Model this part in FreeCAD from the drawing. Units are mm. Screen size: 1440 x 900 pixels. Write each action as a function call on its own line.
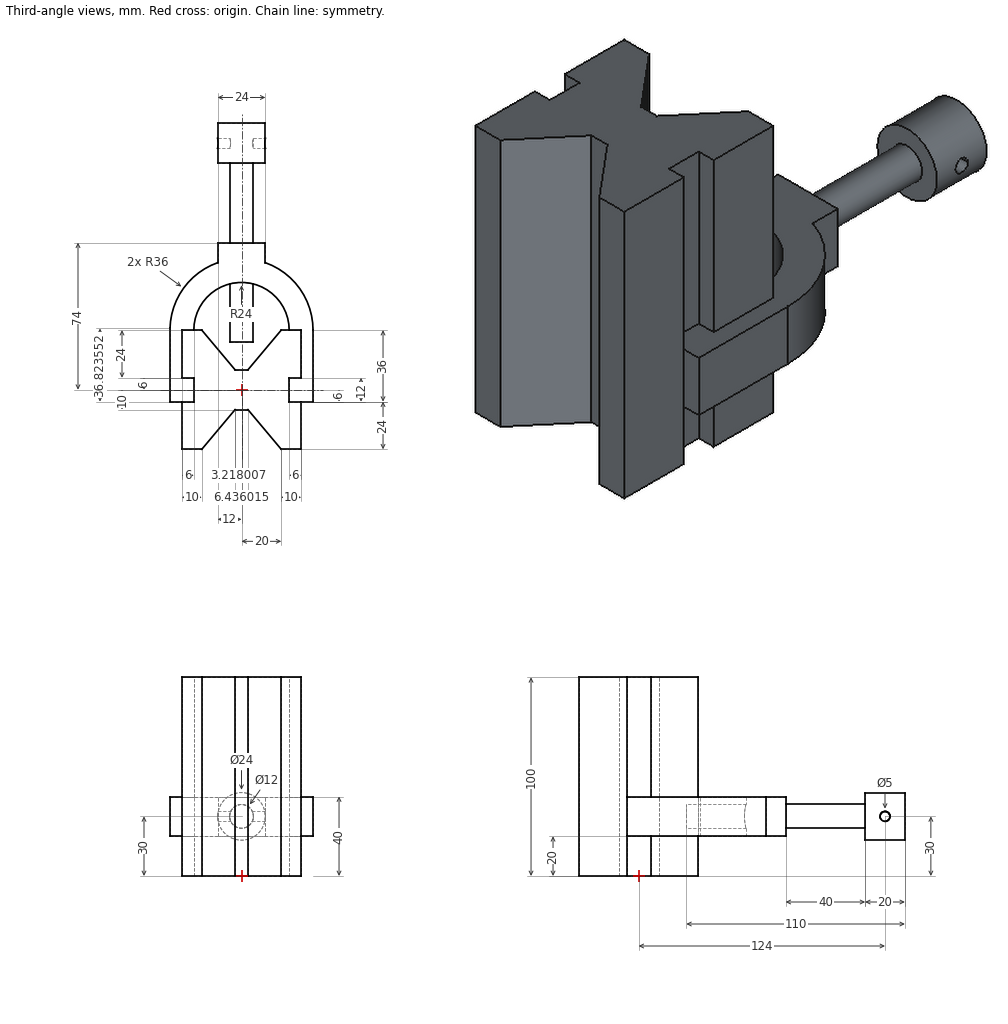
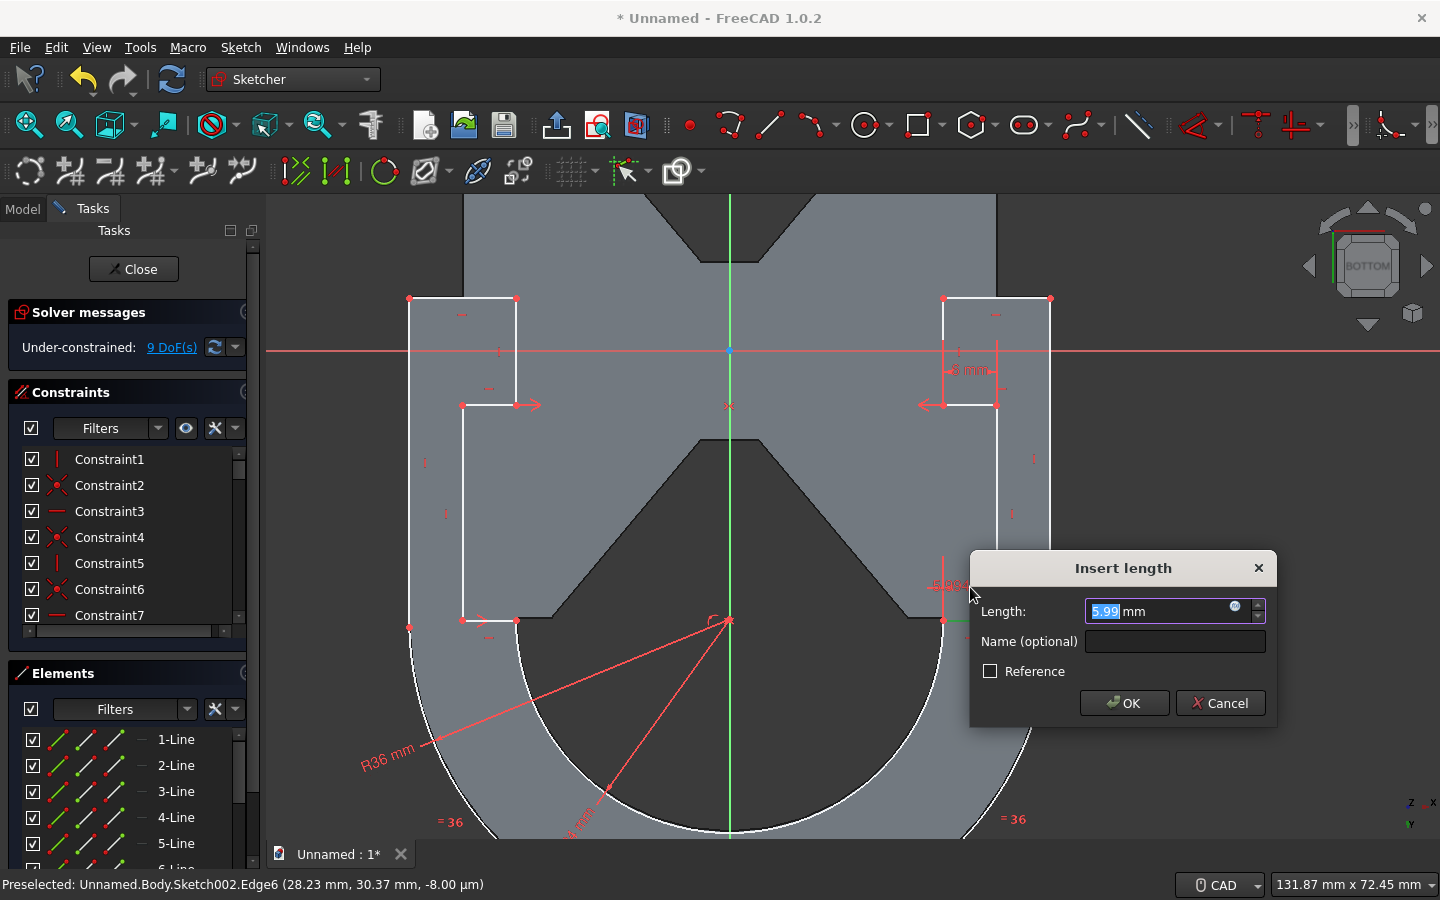
text(6)
key(Return)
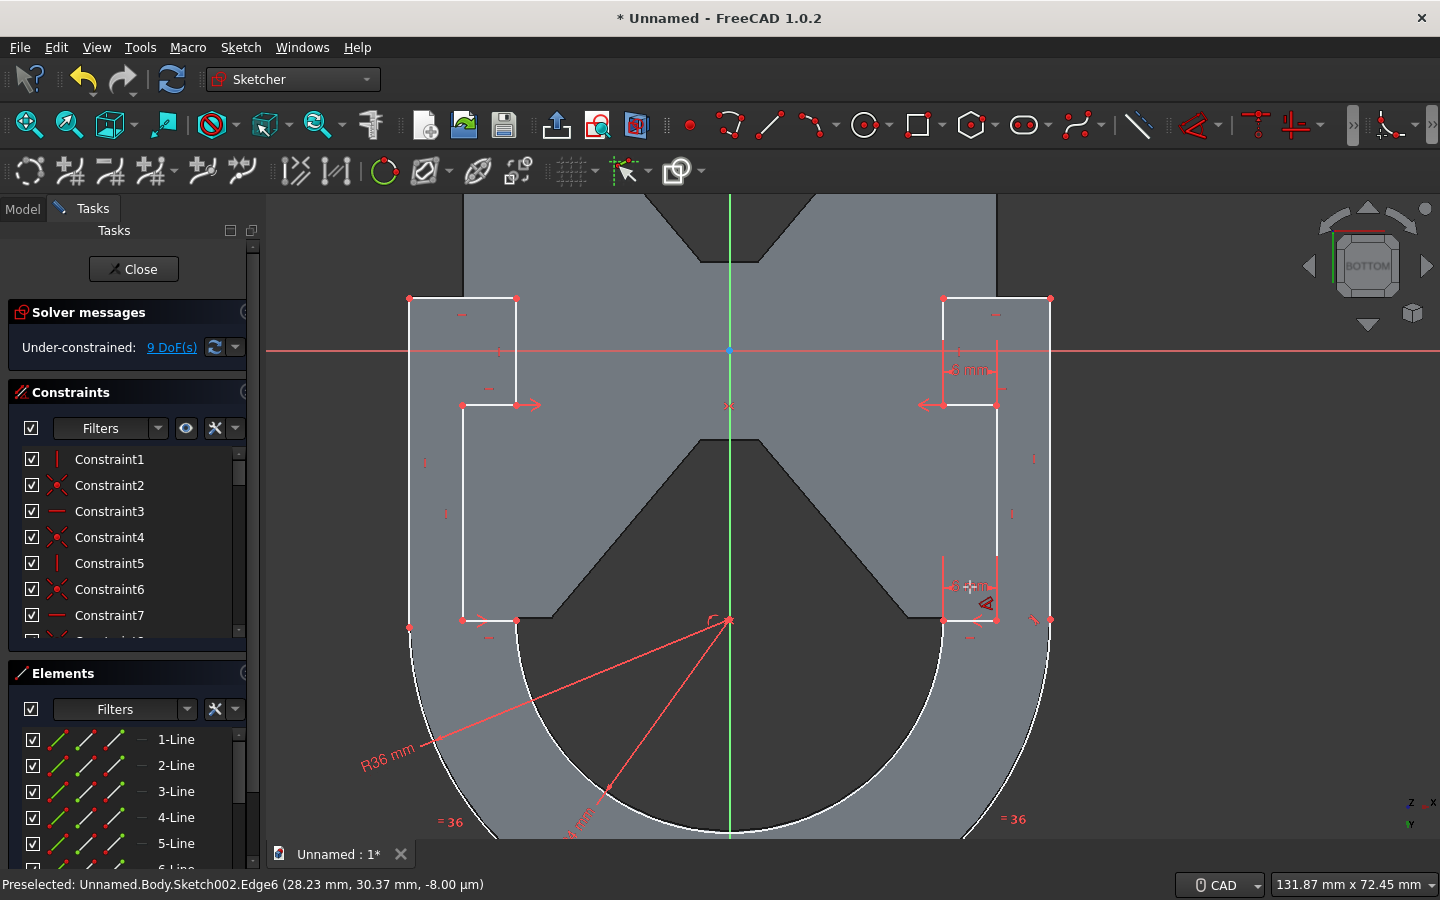
click(1050, 523)
click(1084, 459)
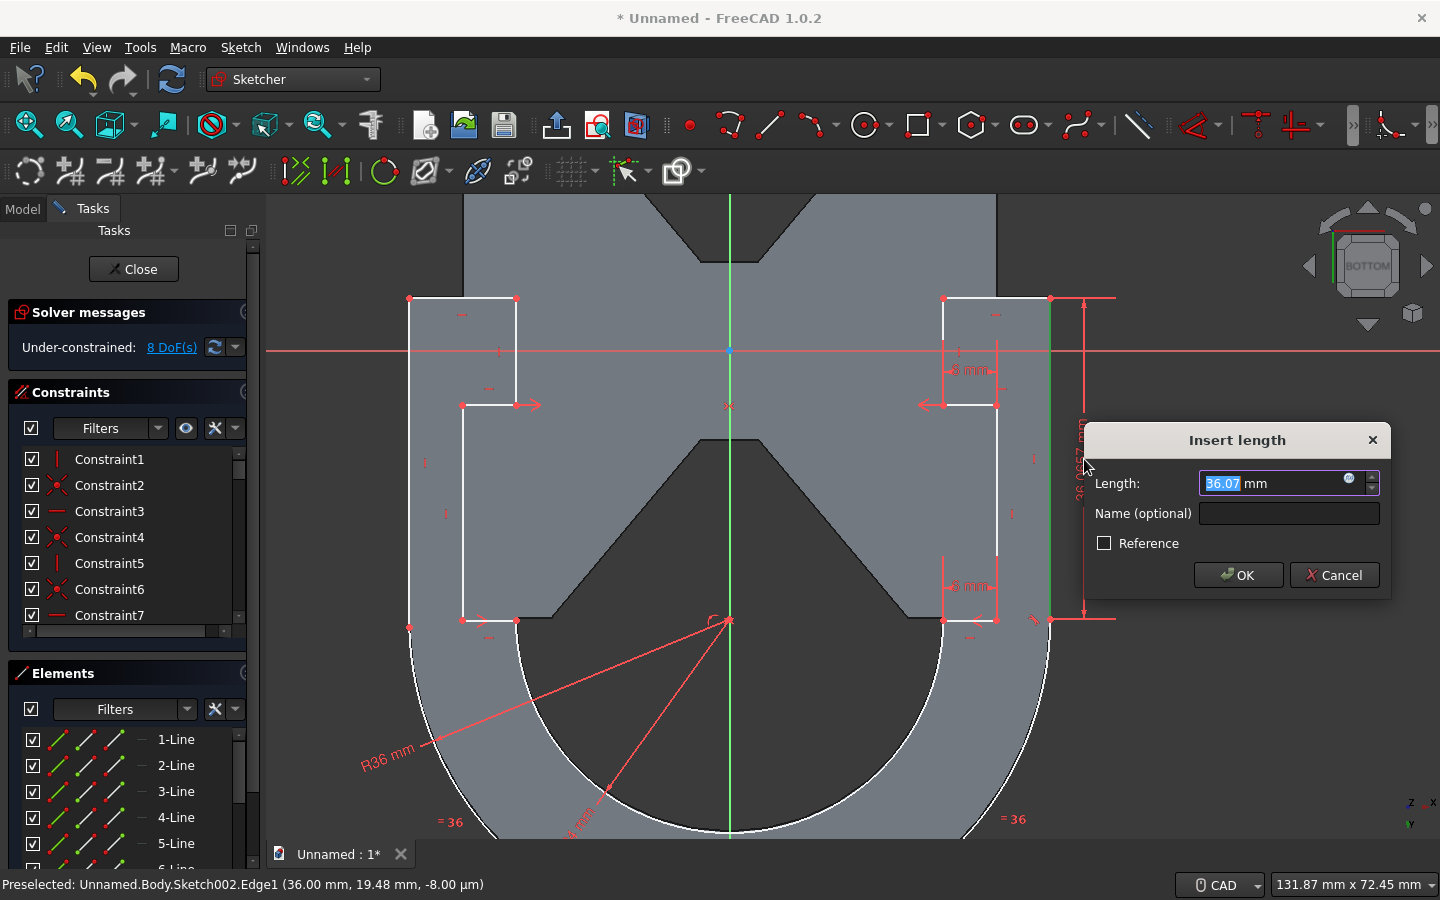
text(36)
key(Return)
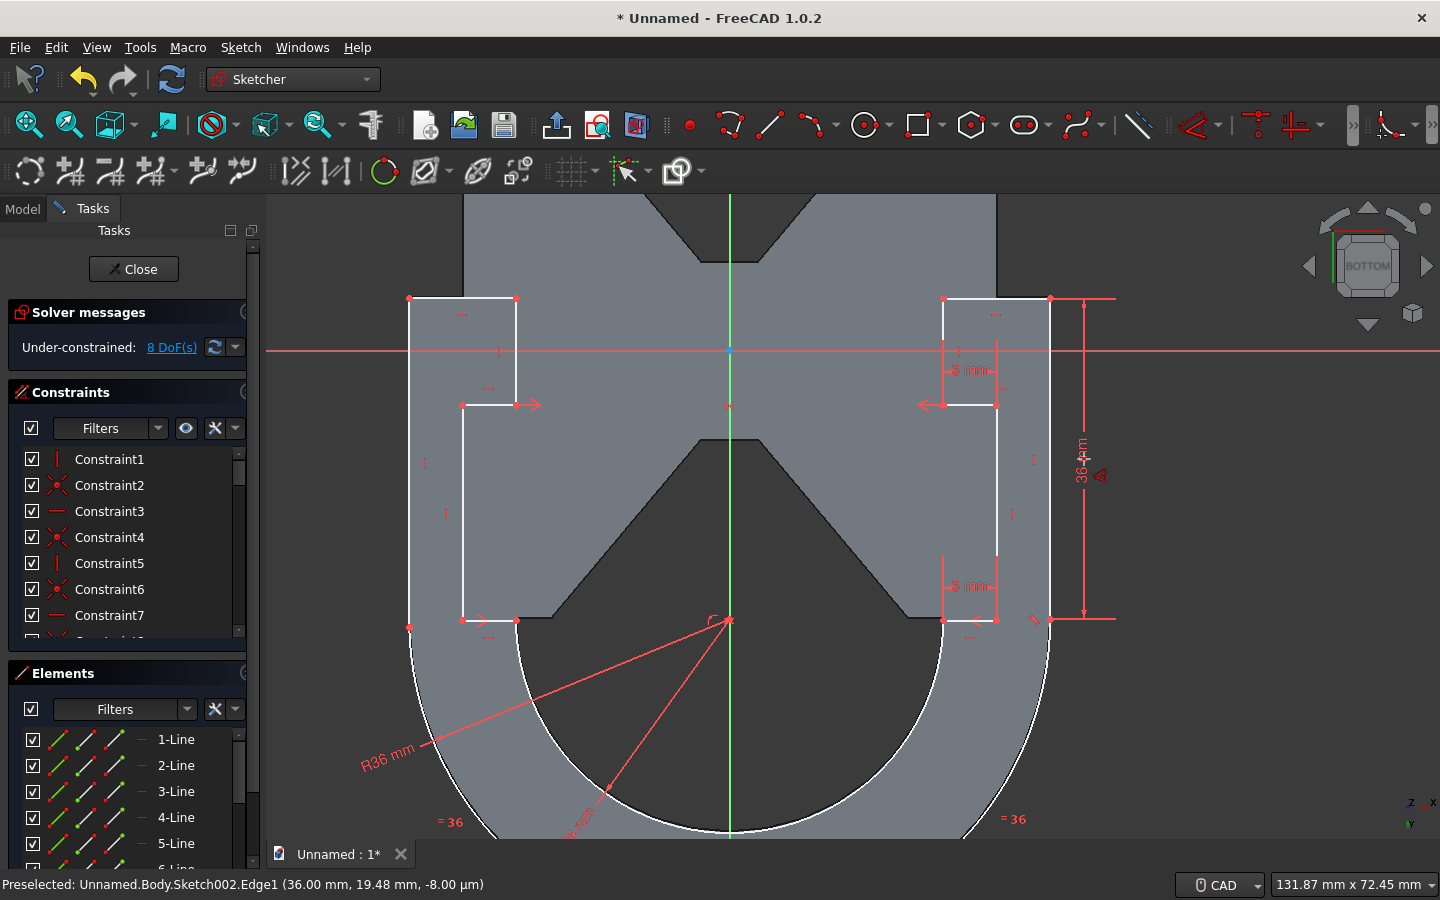
click(943, 331)
click(977, 328)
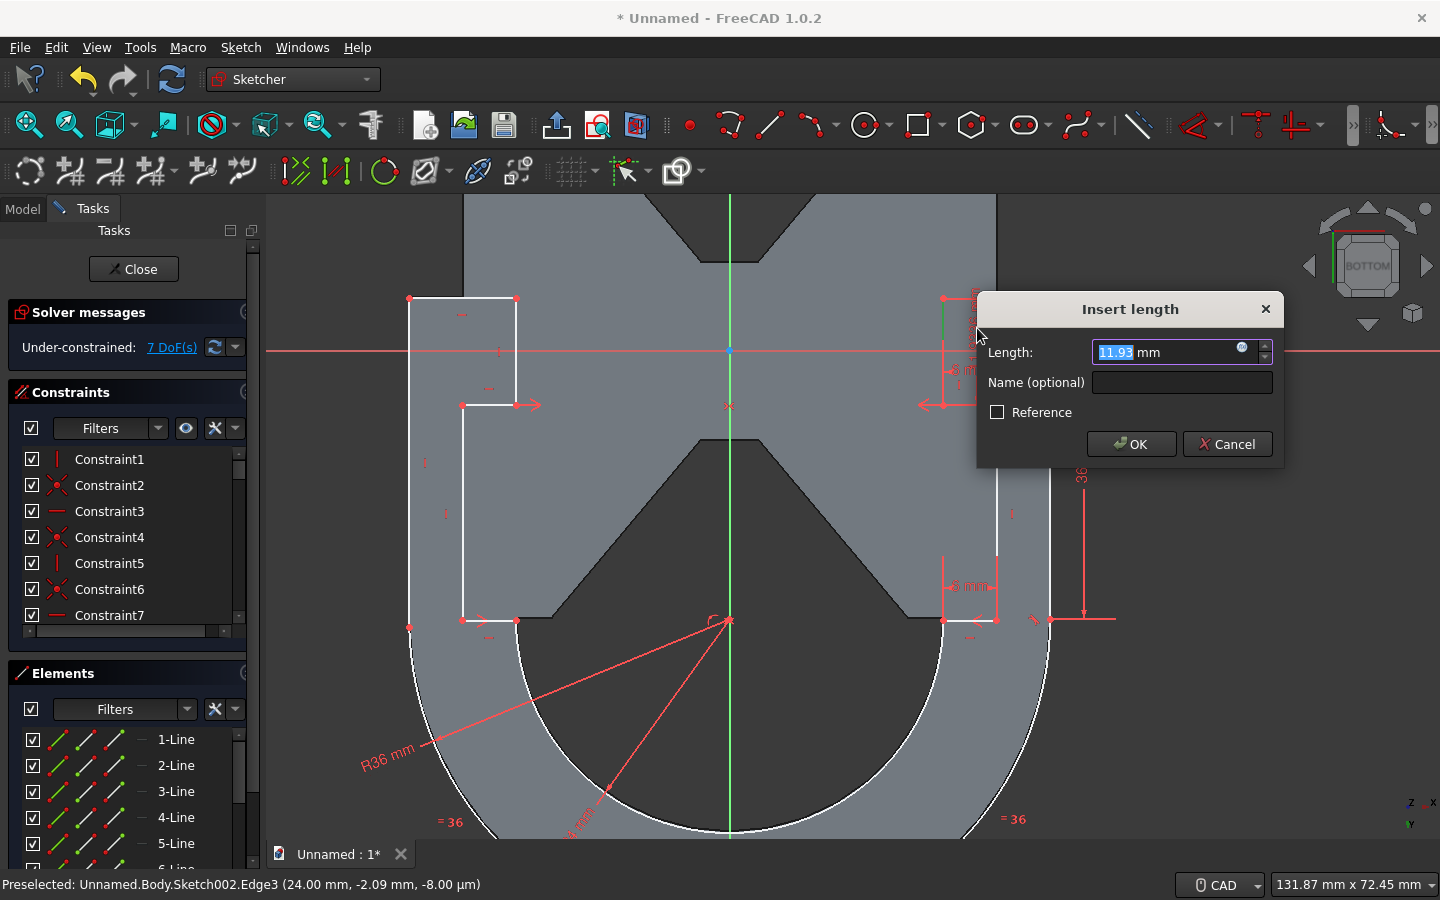
text(12)
key(Return)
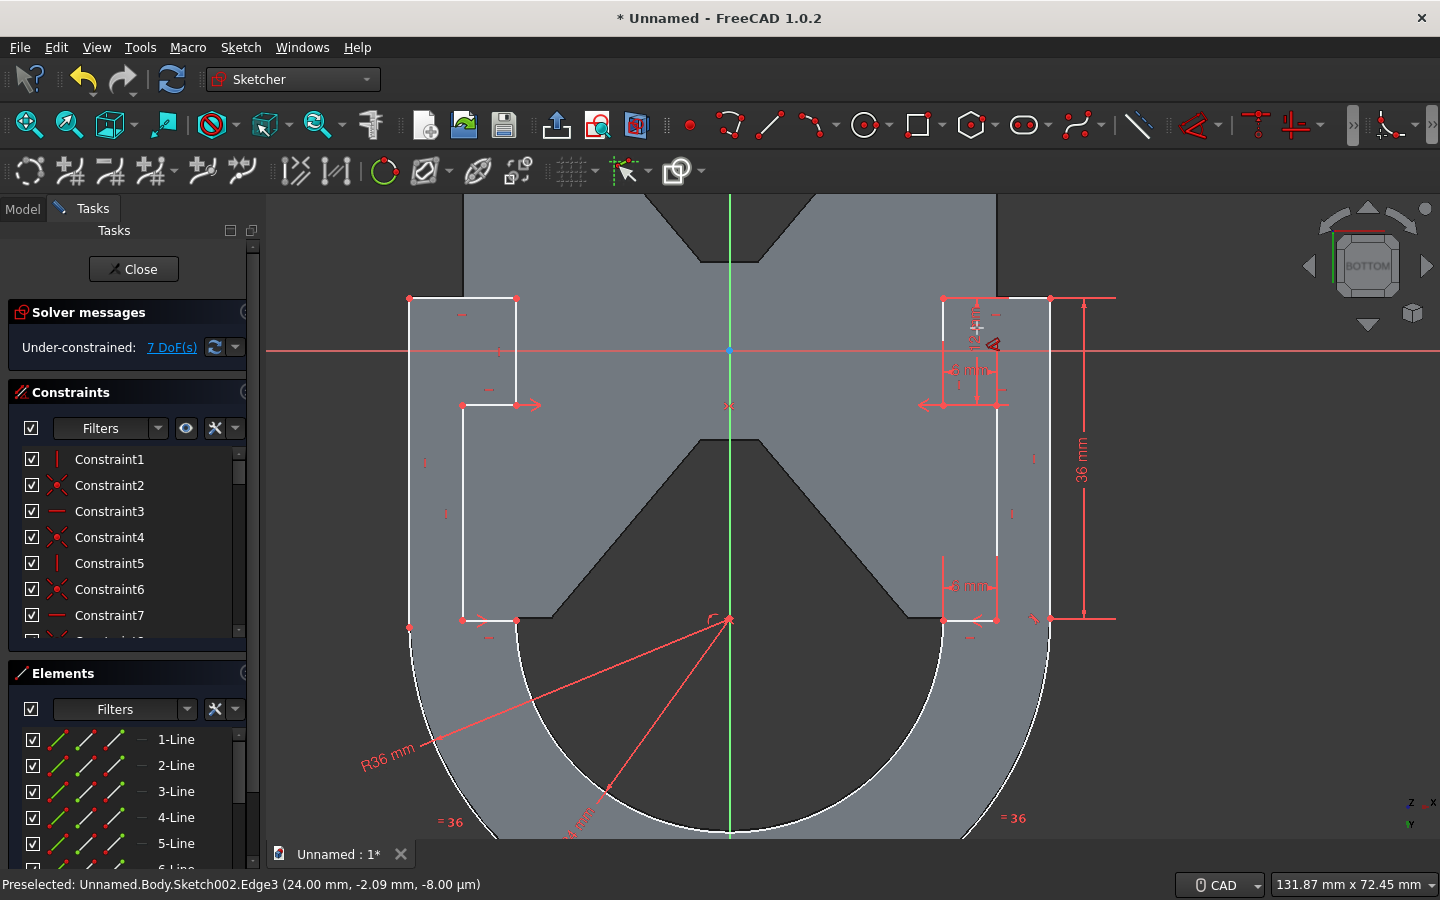
click(997, 470)
click(1031, 513)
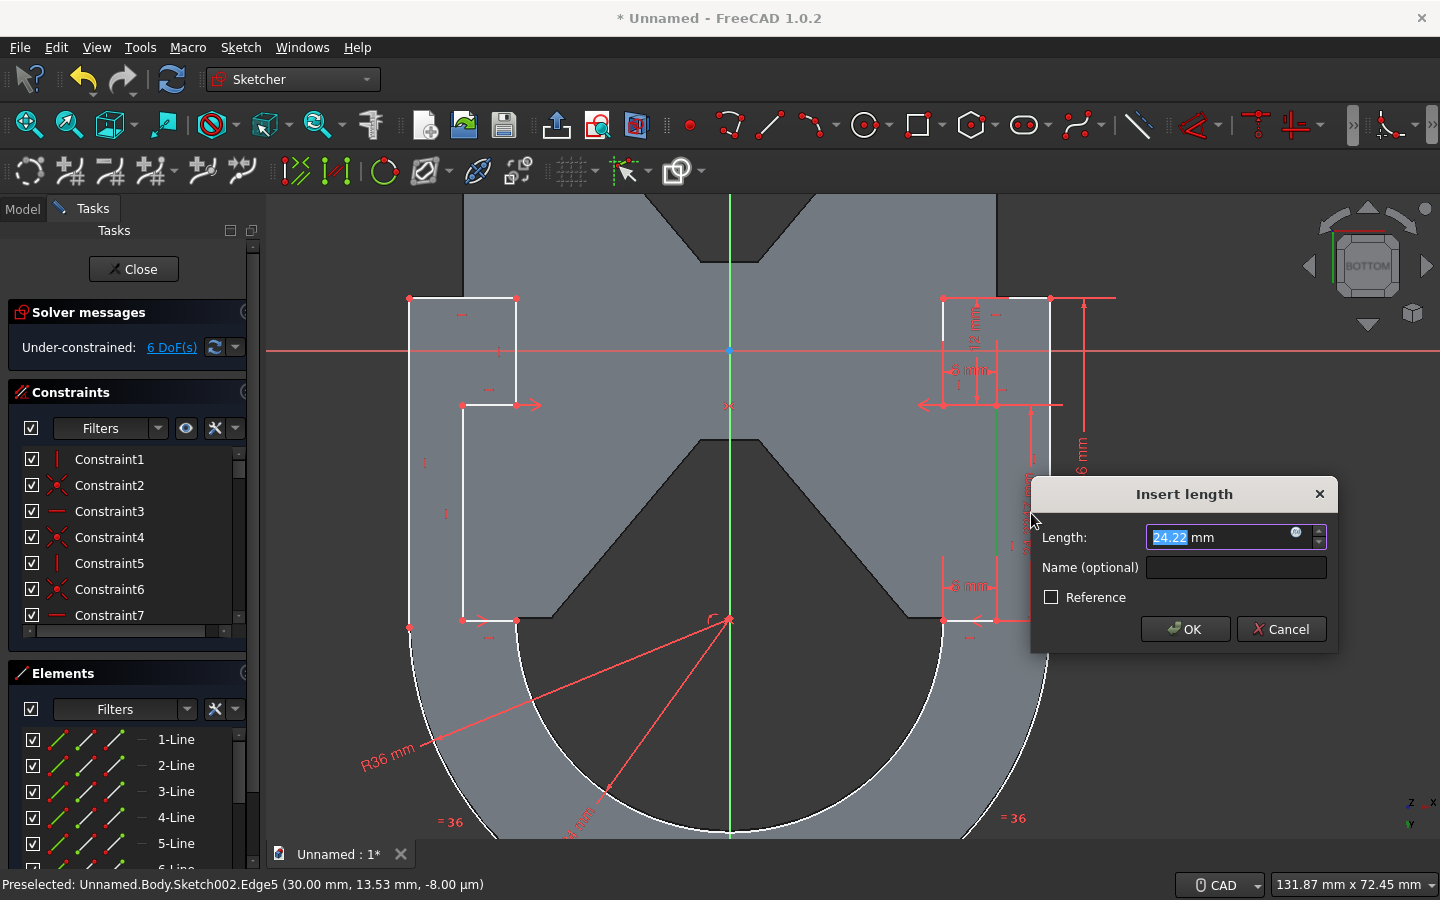
text(24)
key(Return)